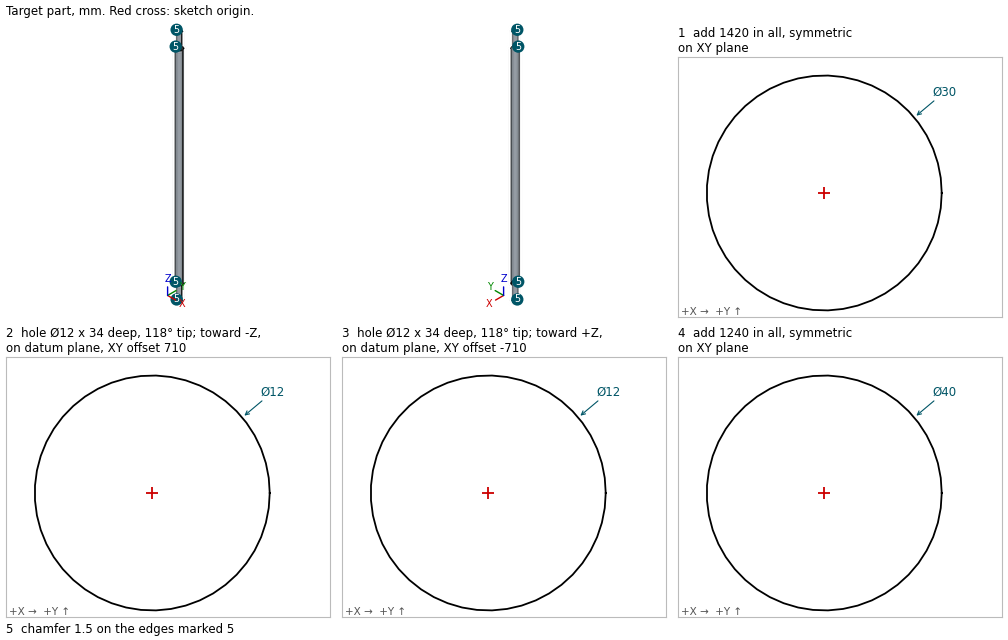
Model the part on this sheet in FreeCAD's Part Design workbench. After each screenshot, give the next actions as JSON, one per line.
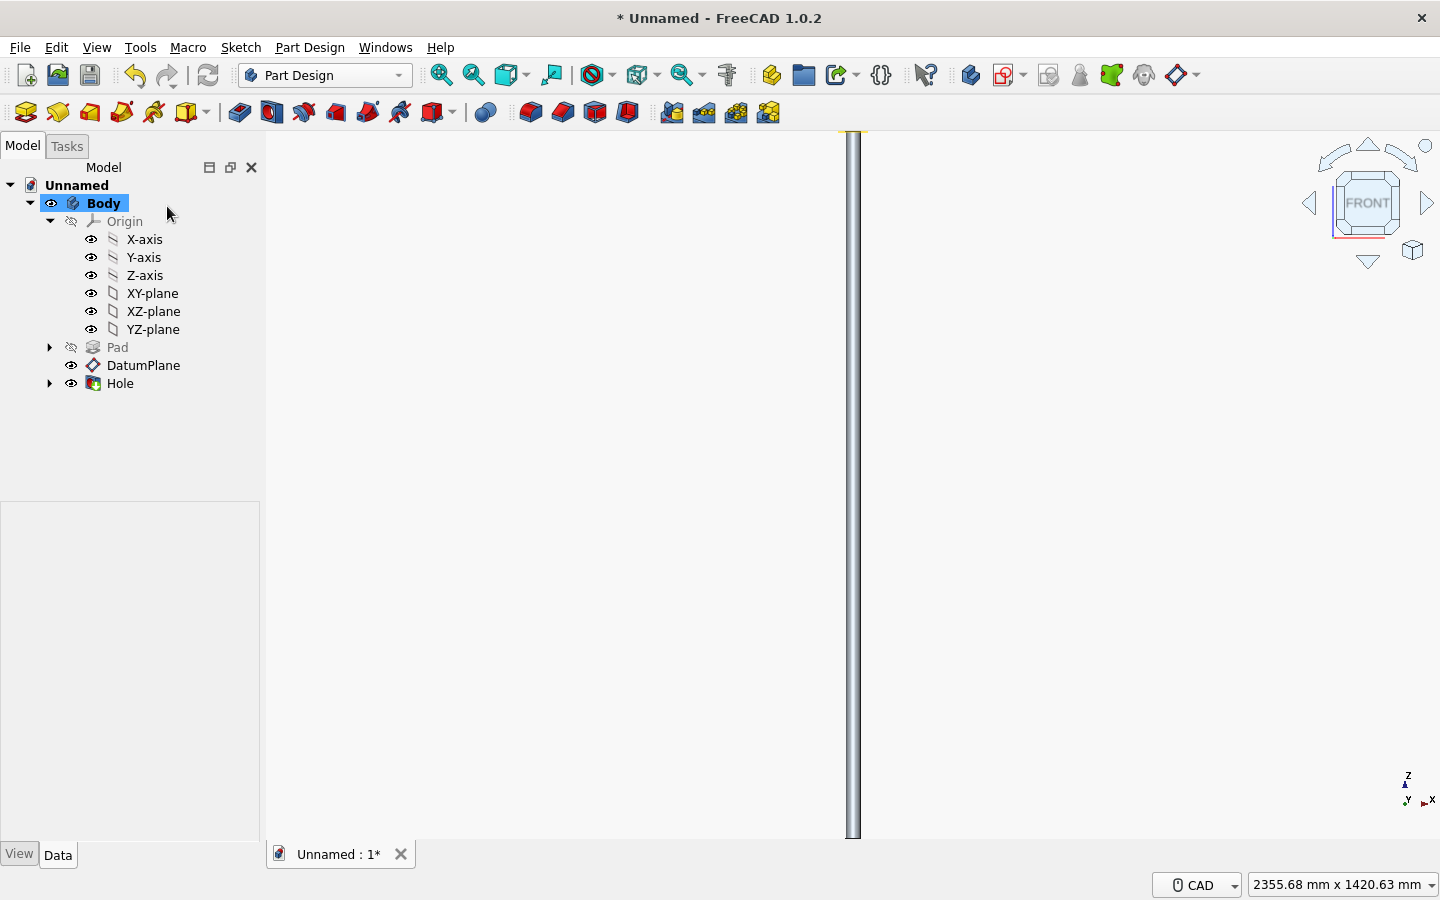
{"action": "left_click", "coordinate": [116, 365]}
{"action": "key", "text": "space"}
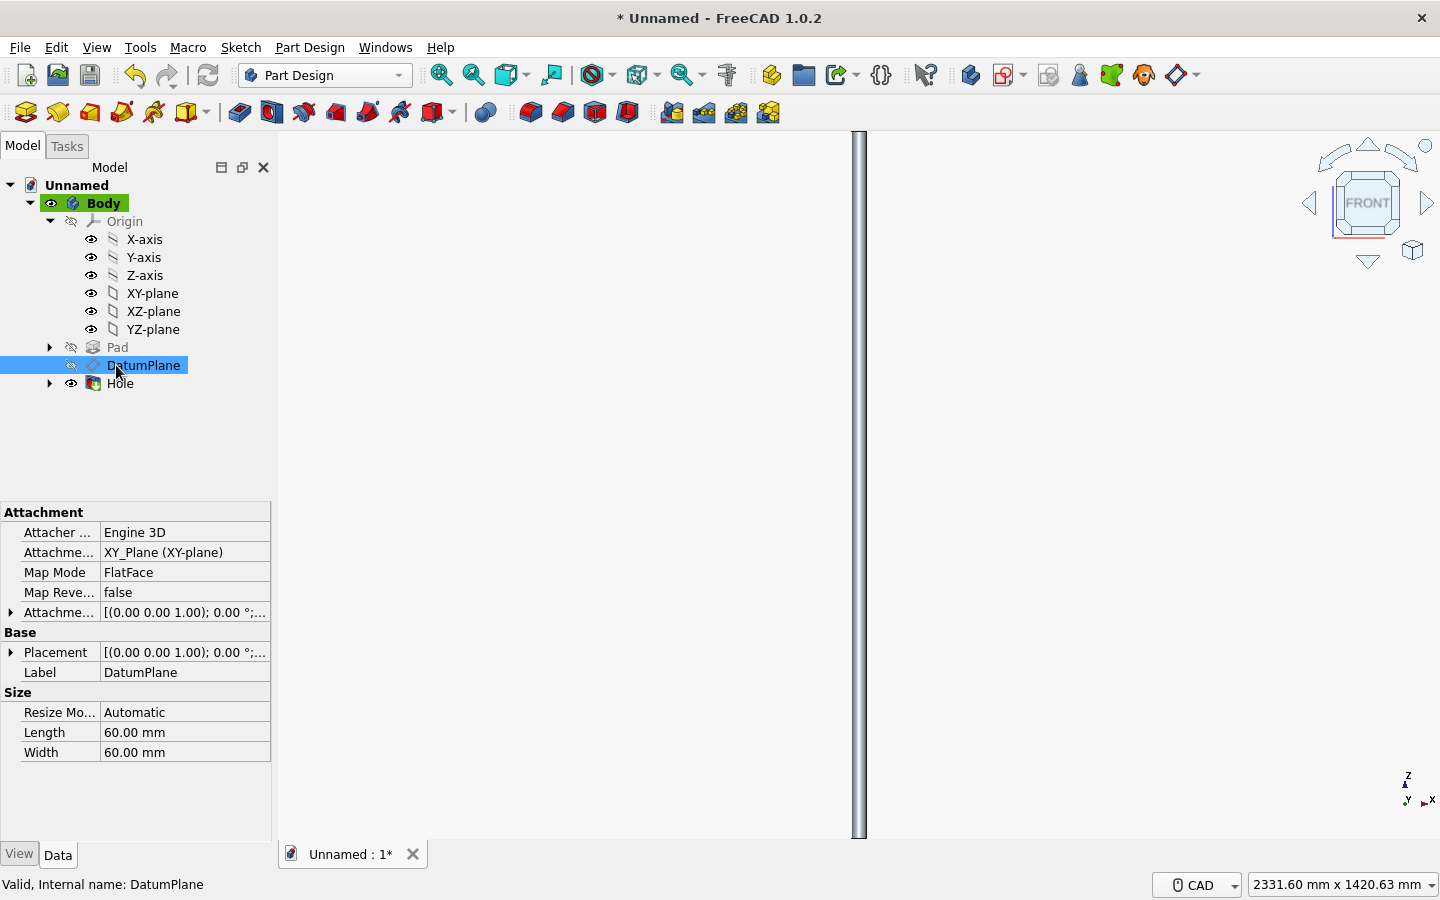
{"action": "left_click", "coordinate": [442, 76]}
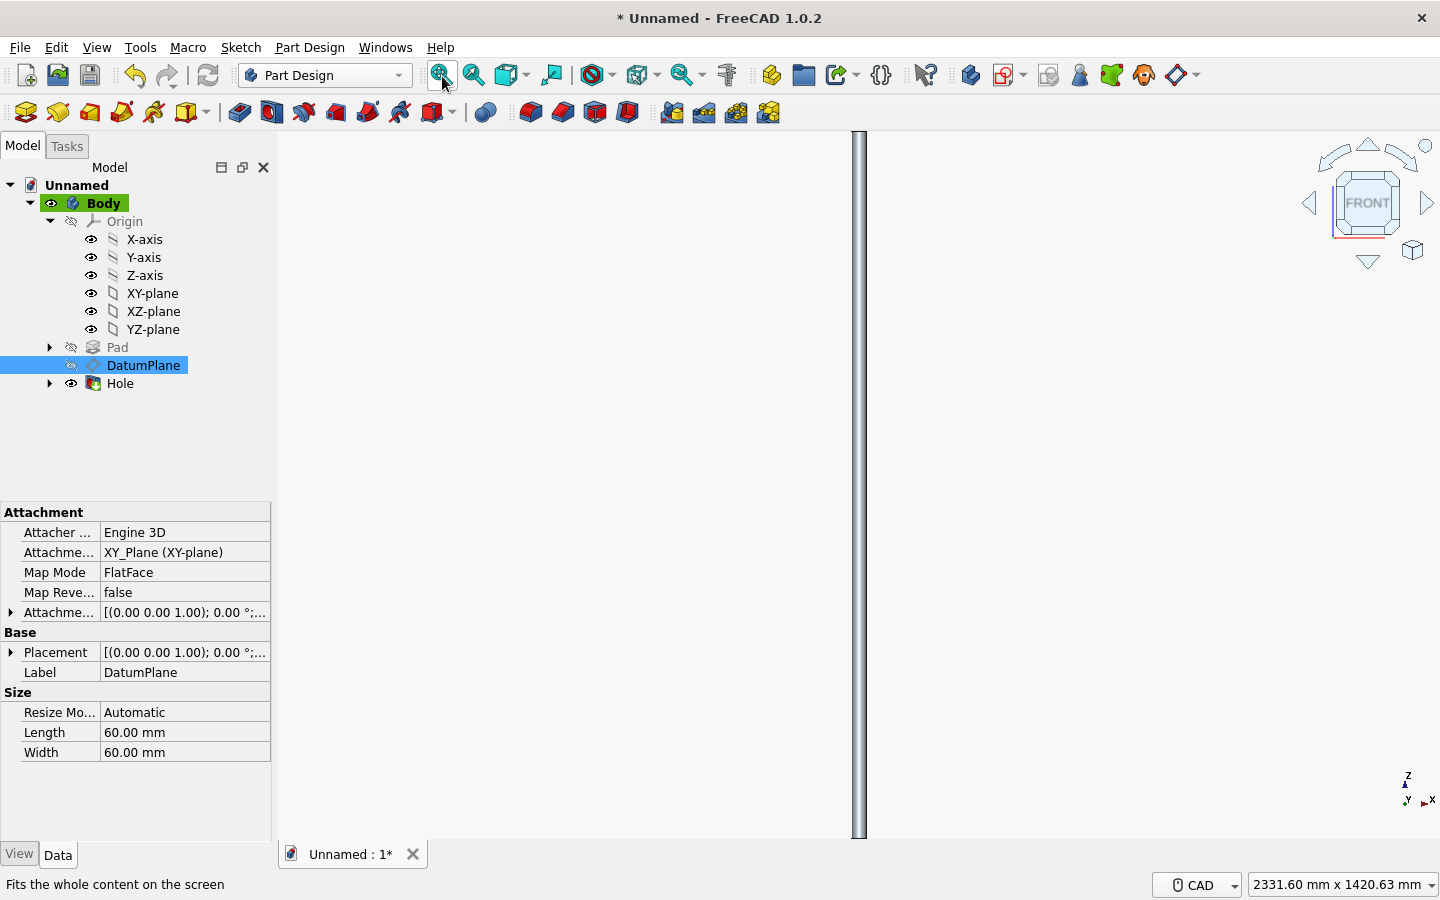
{"action": "key", "text": "5"}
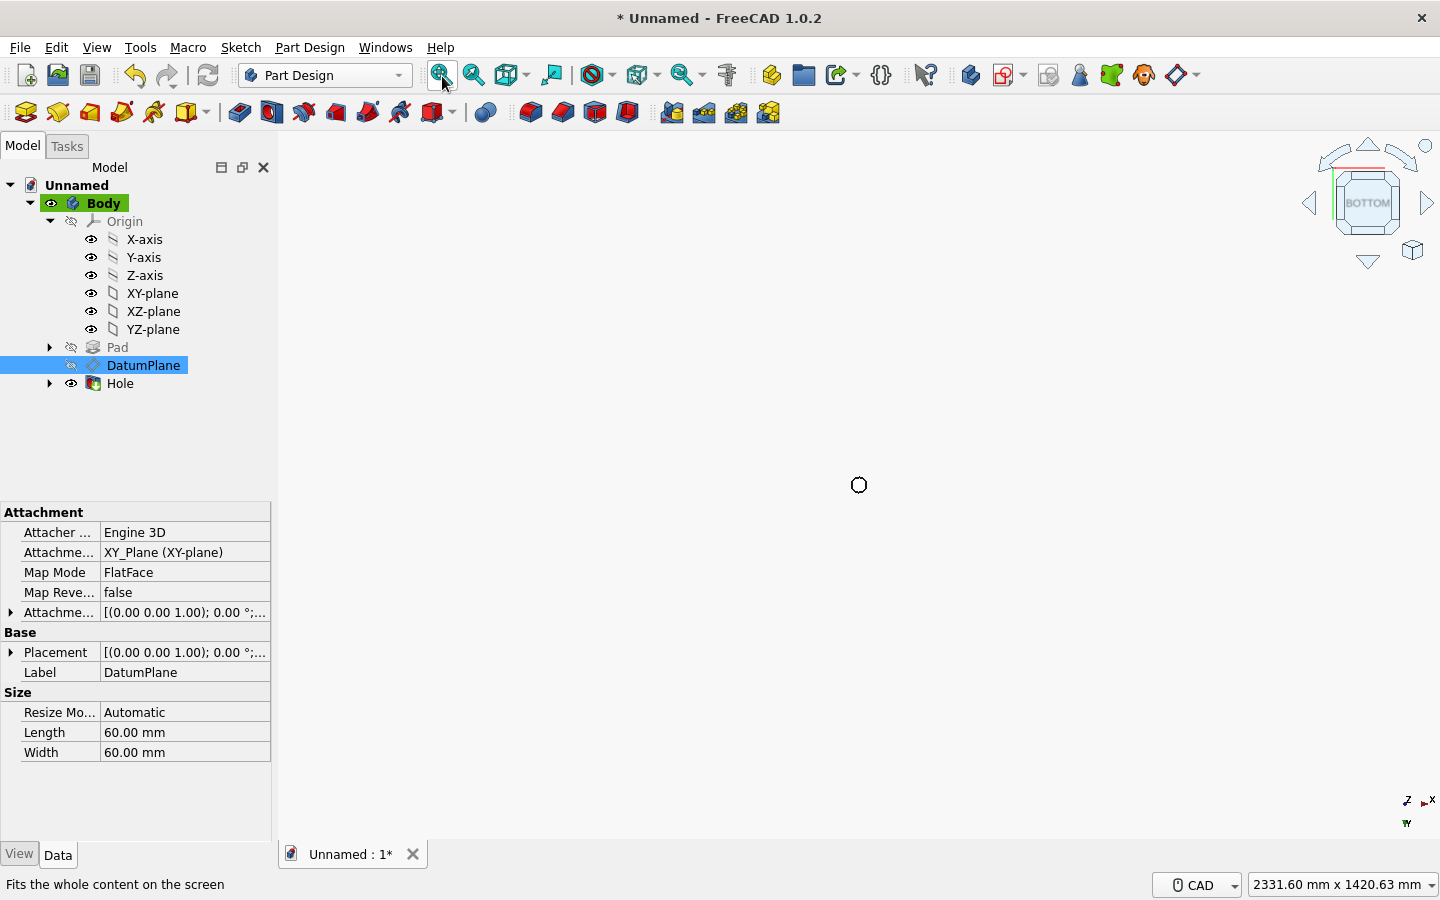
{"action": "left_click", "coordinate": [442, 76]}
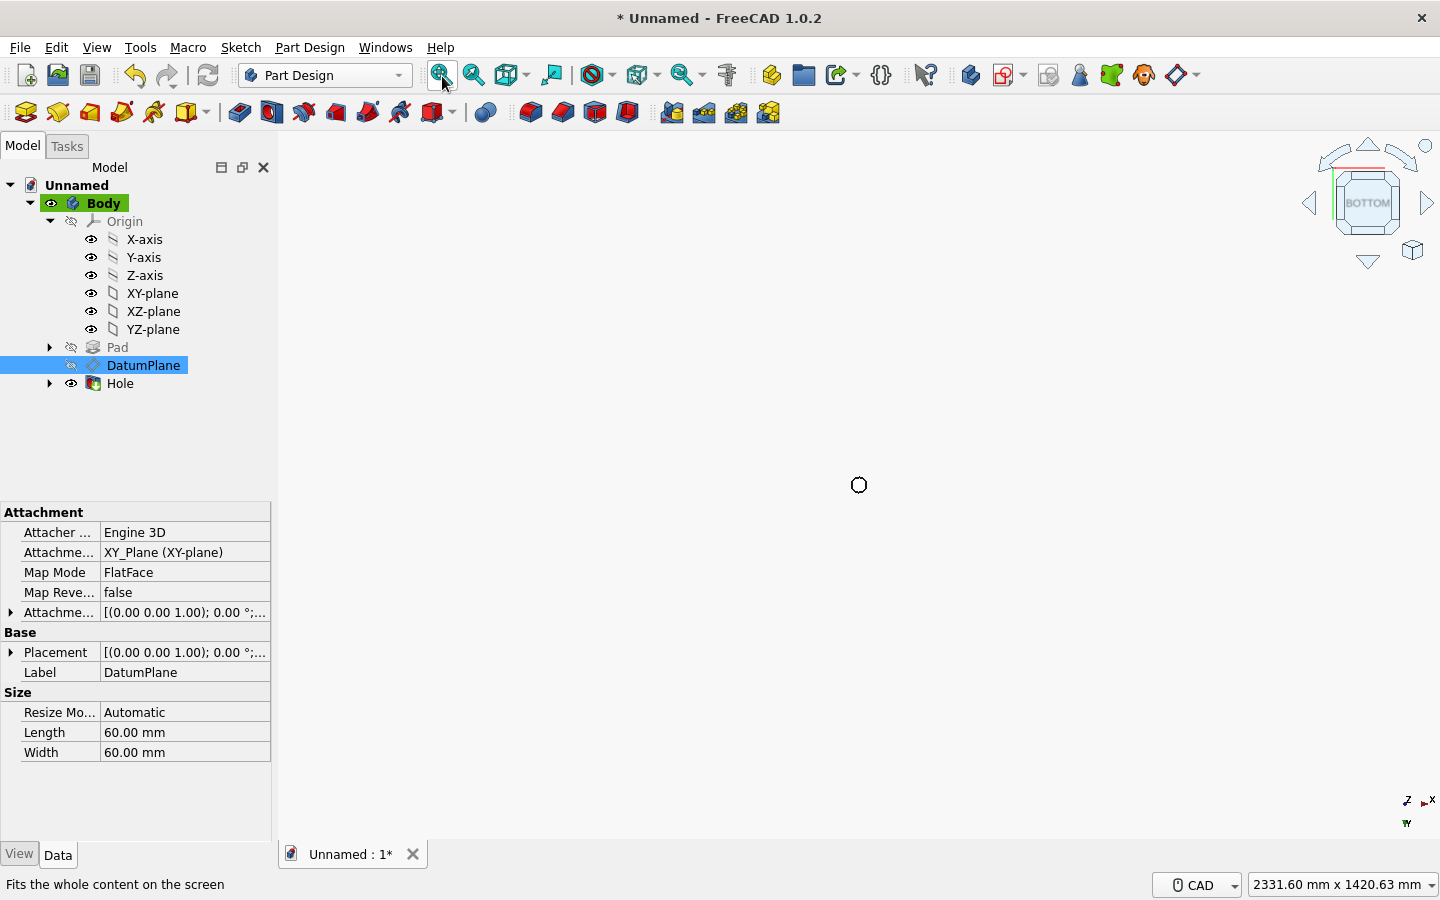
{"action": "key", "text": "1"}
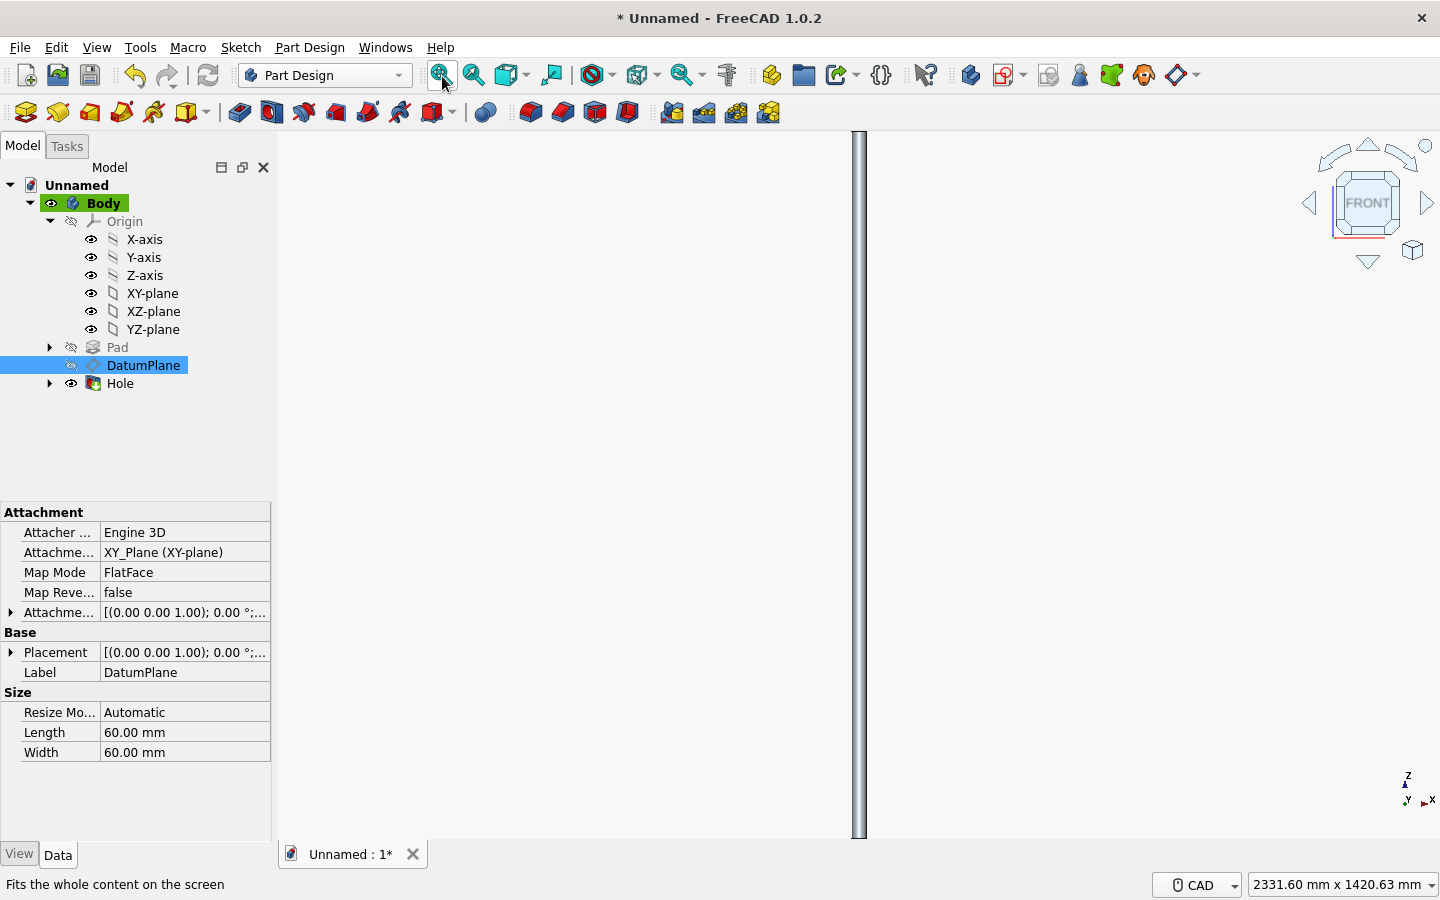
{"action": "left_click", "coordinate": [442, 76]}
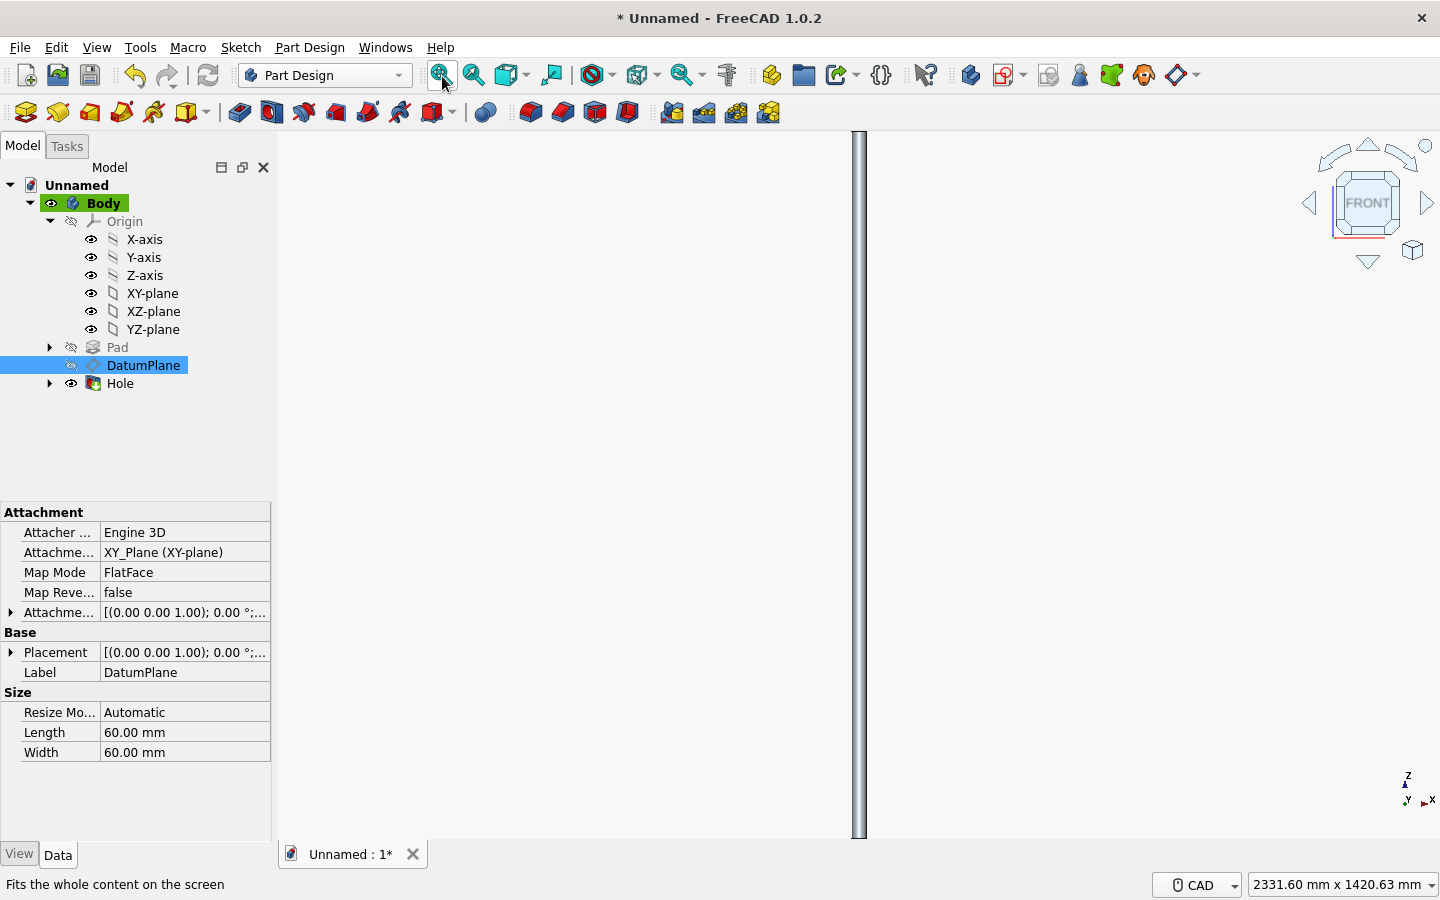
{"action": "key", "text": "3"}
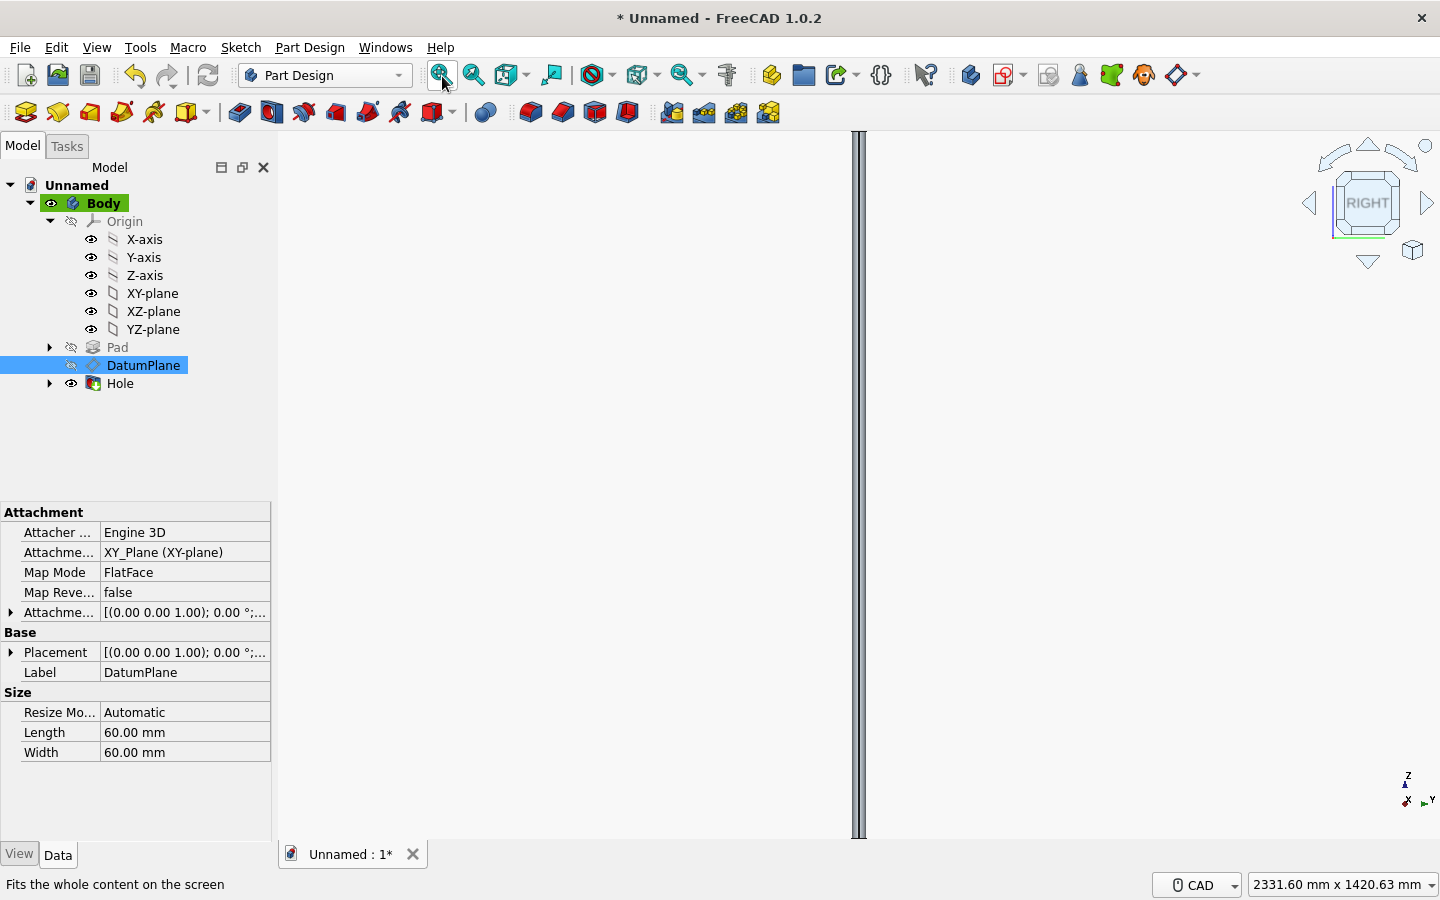
{"action": "left_click", "coordinate": [442, 76]}